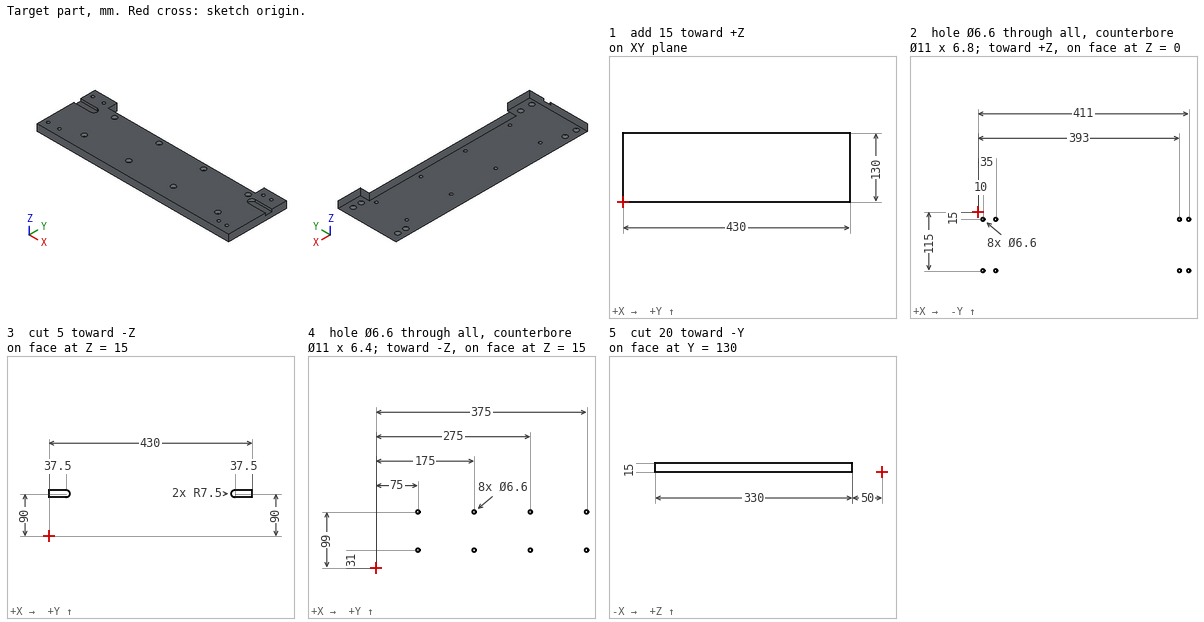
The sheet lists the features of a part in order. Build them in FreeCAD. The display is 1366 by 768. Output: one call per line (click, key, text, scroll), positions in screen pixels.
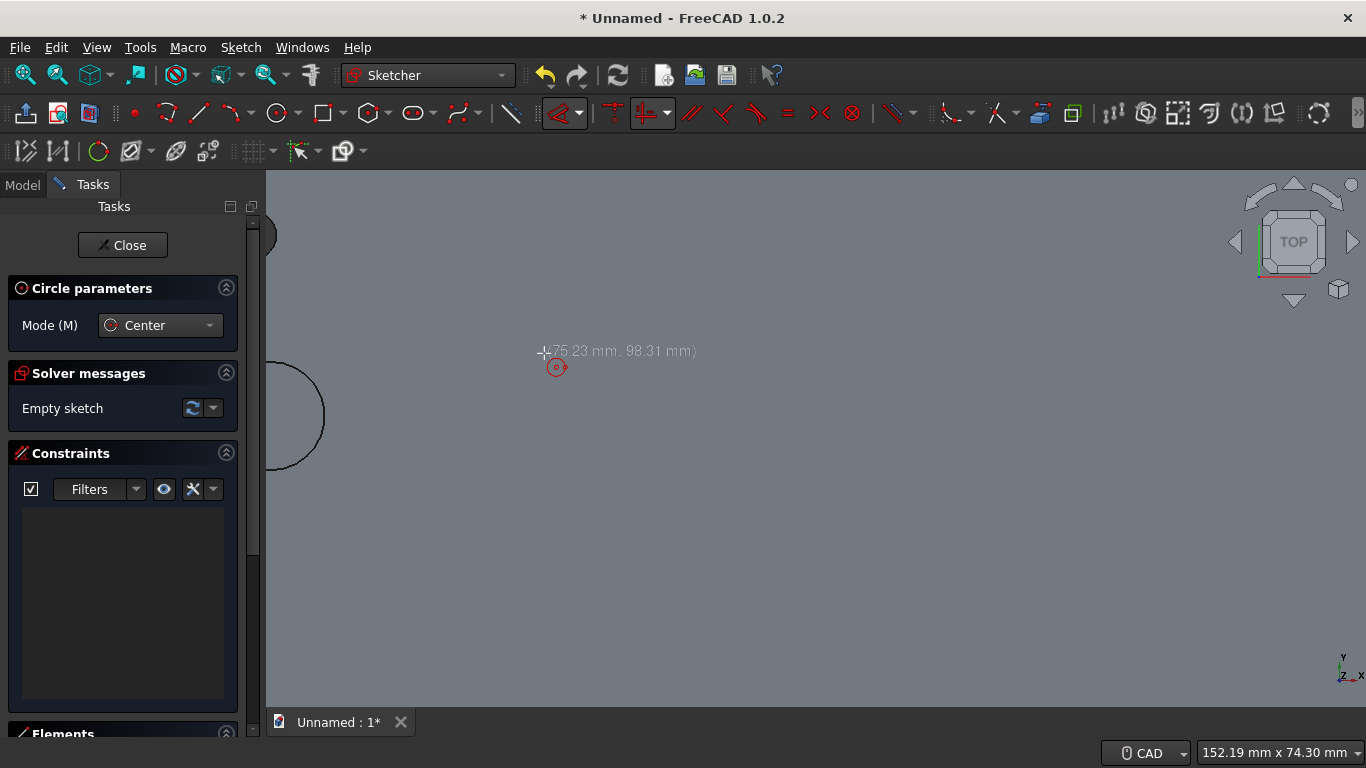
scroll(545, 354, down, 7)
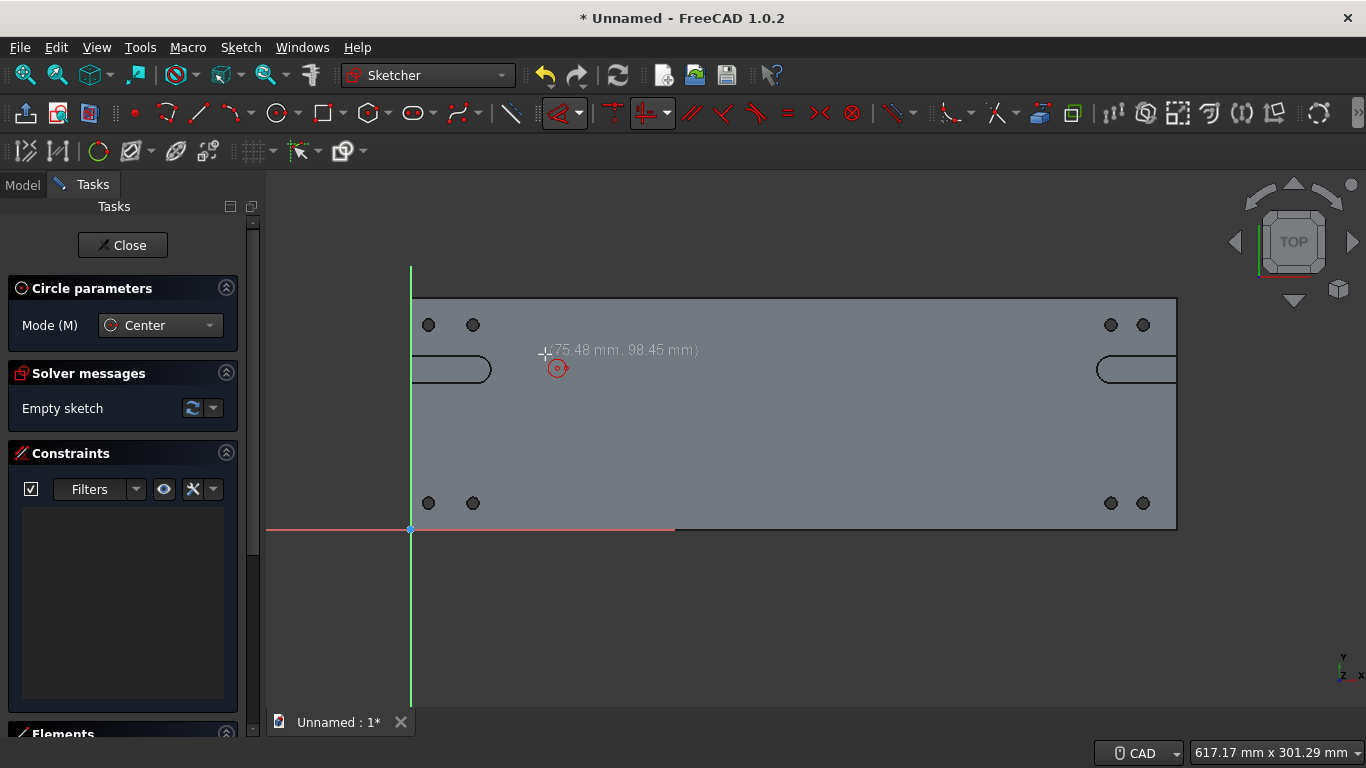
click(544, 354)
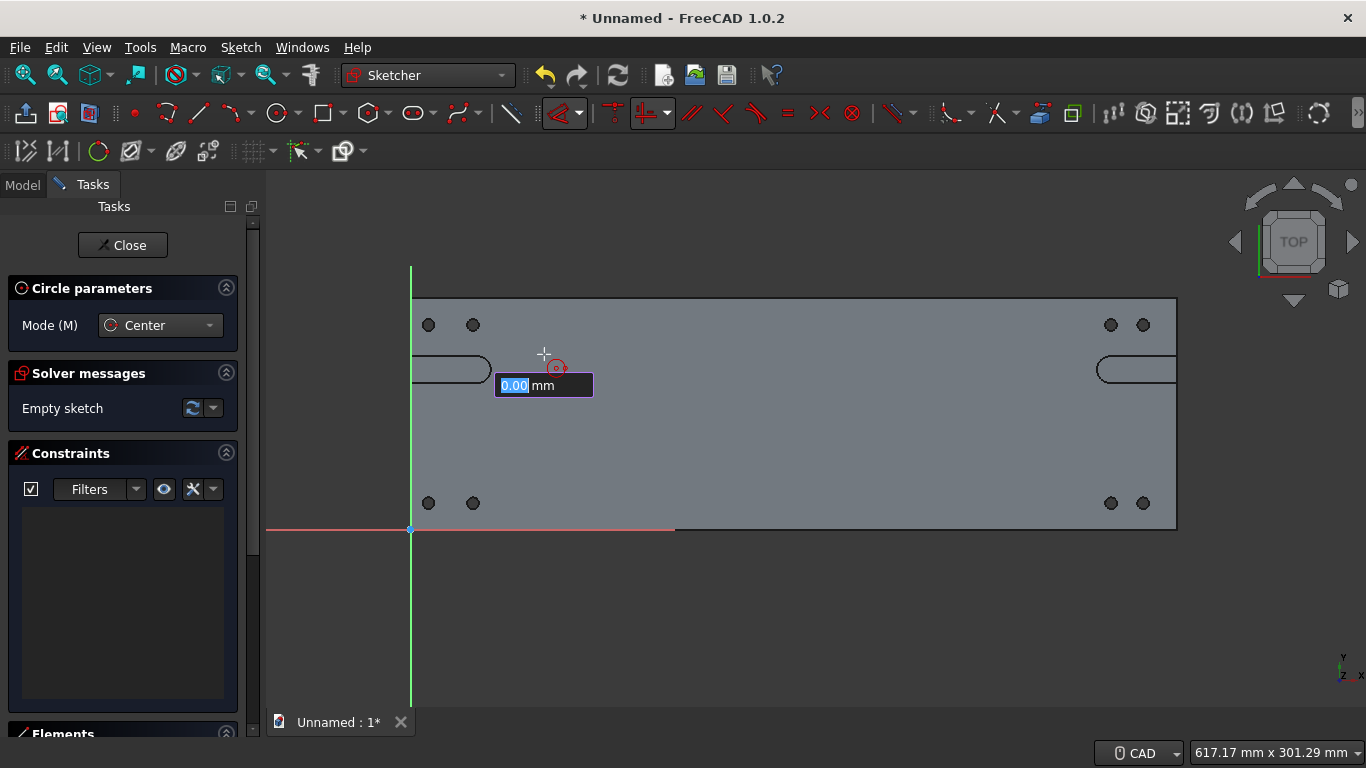
scroll(548, 349, up, 5)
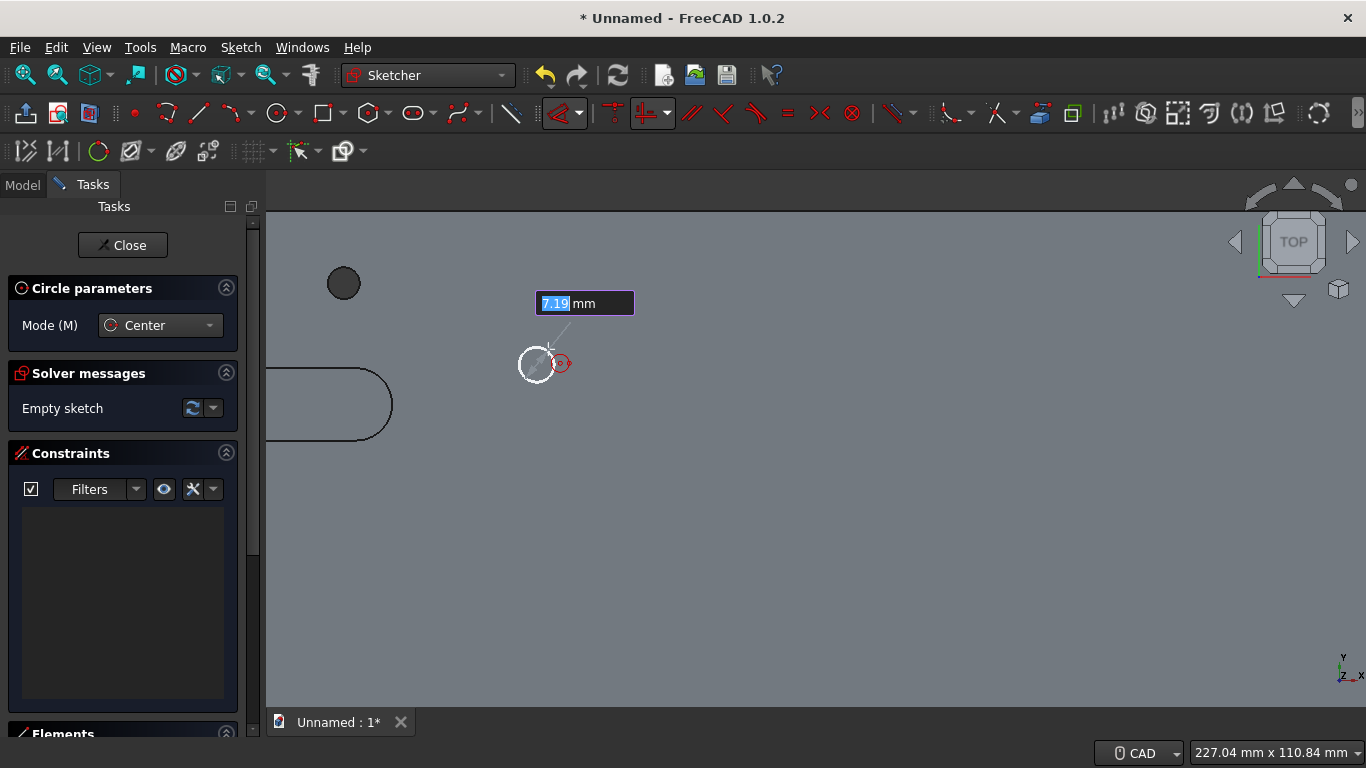
click(549, 349)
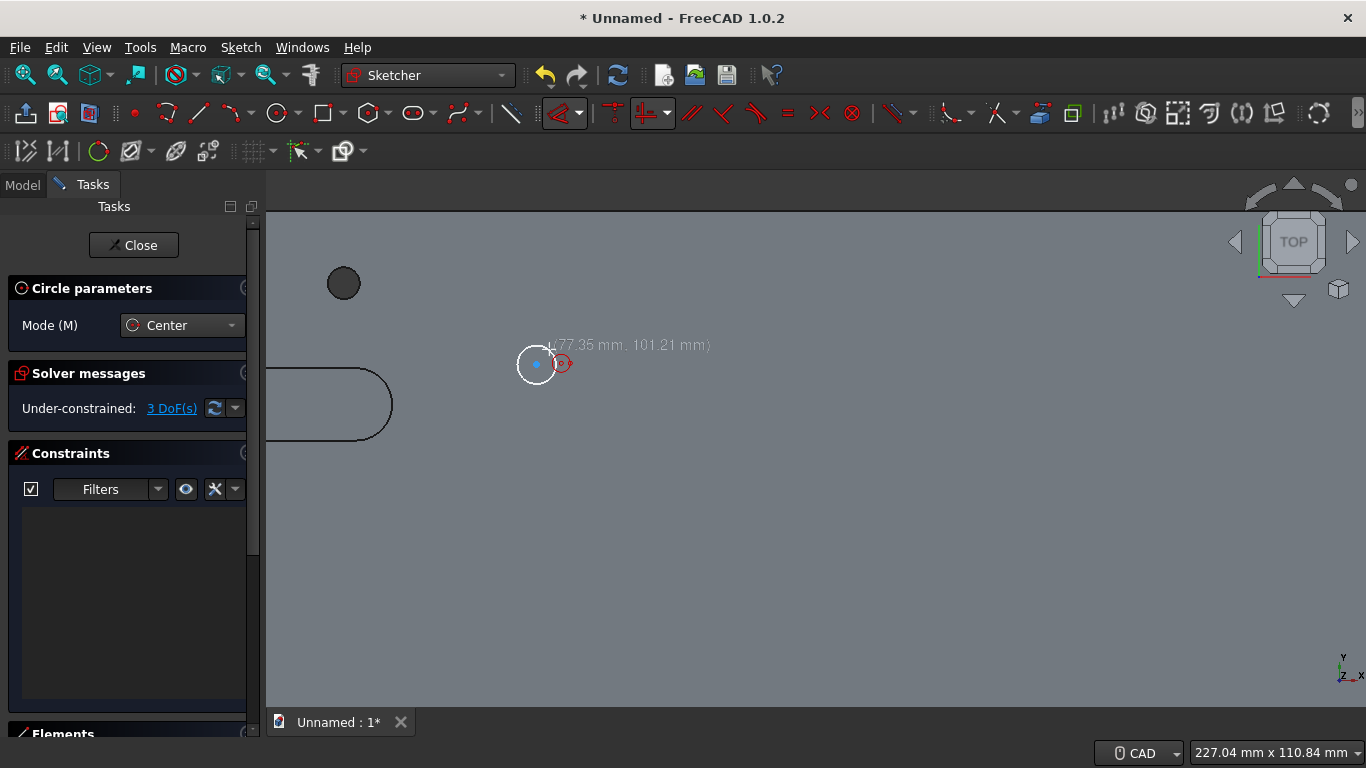
scroll(1022, 361, up, 2)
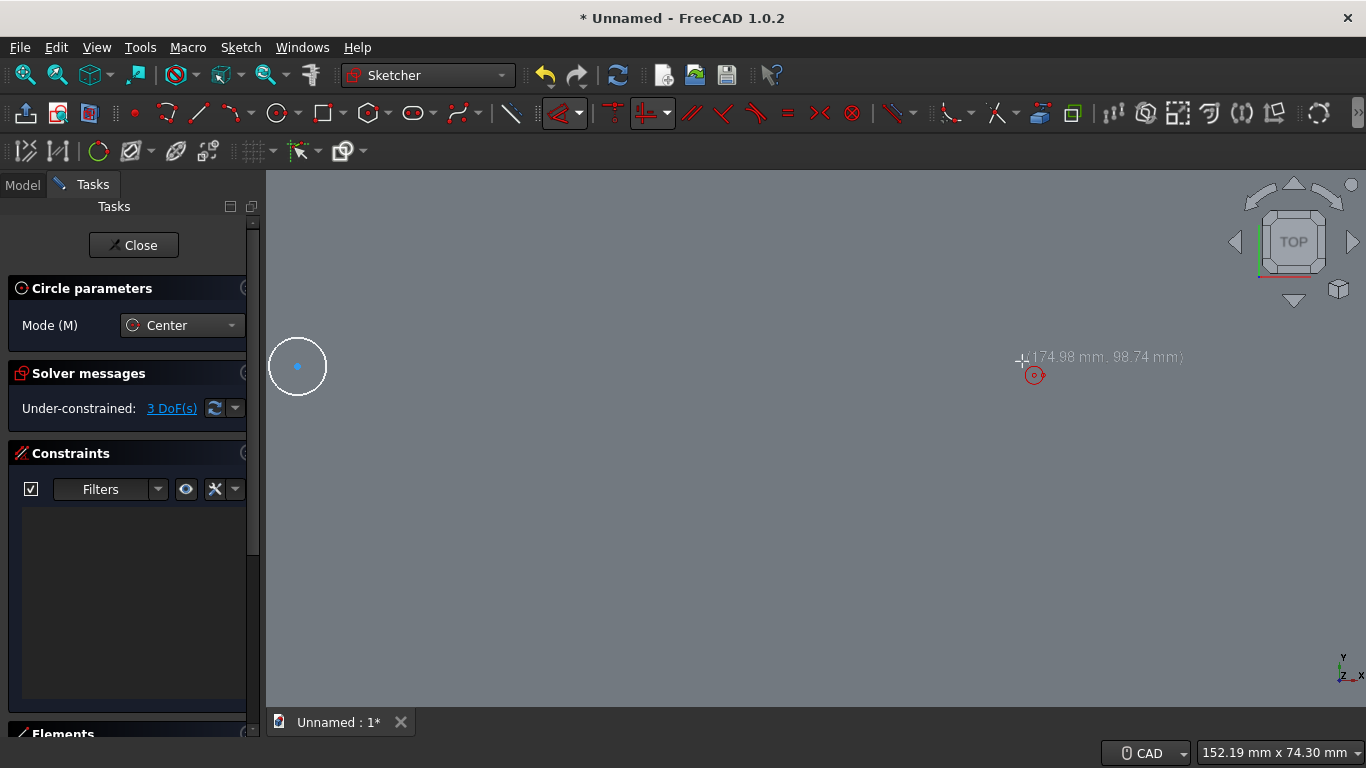
scroll(624, 351, down, 7)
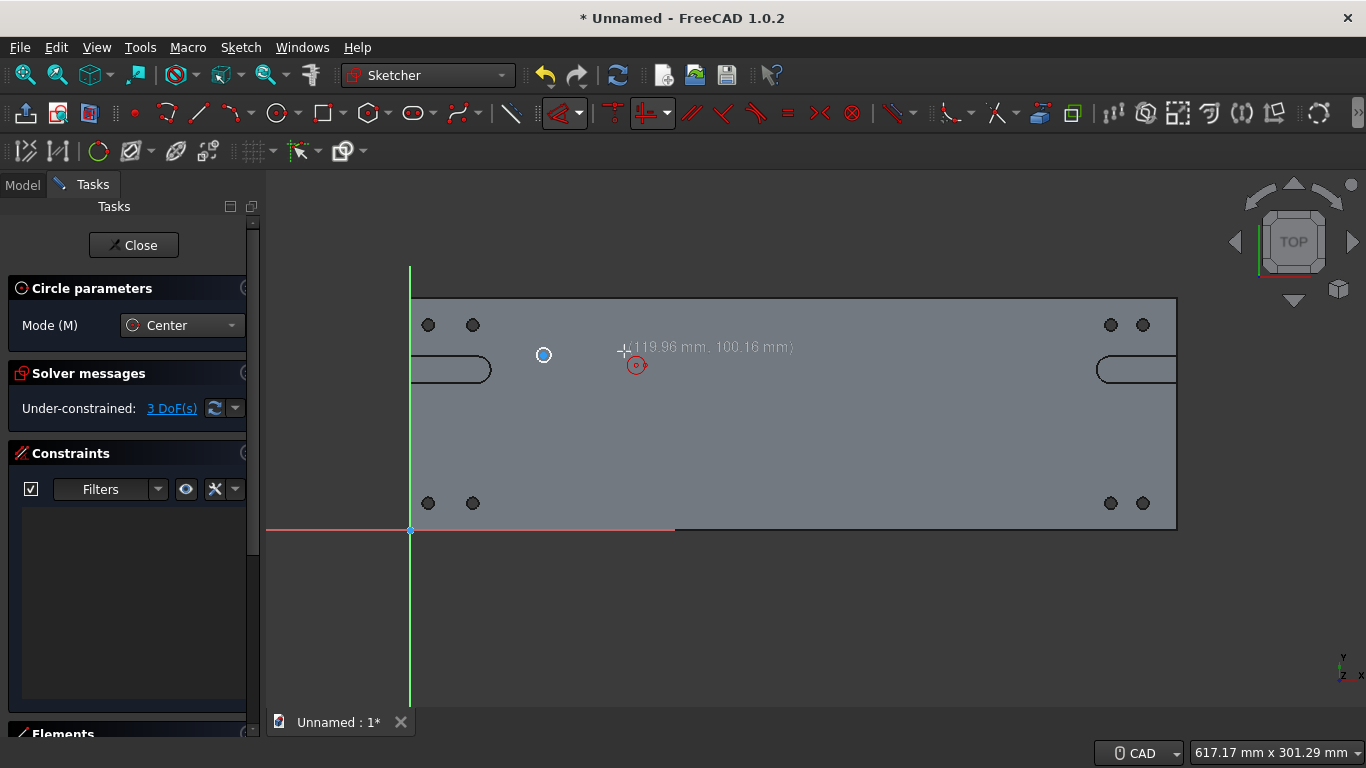
click(722, 354)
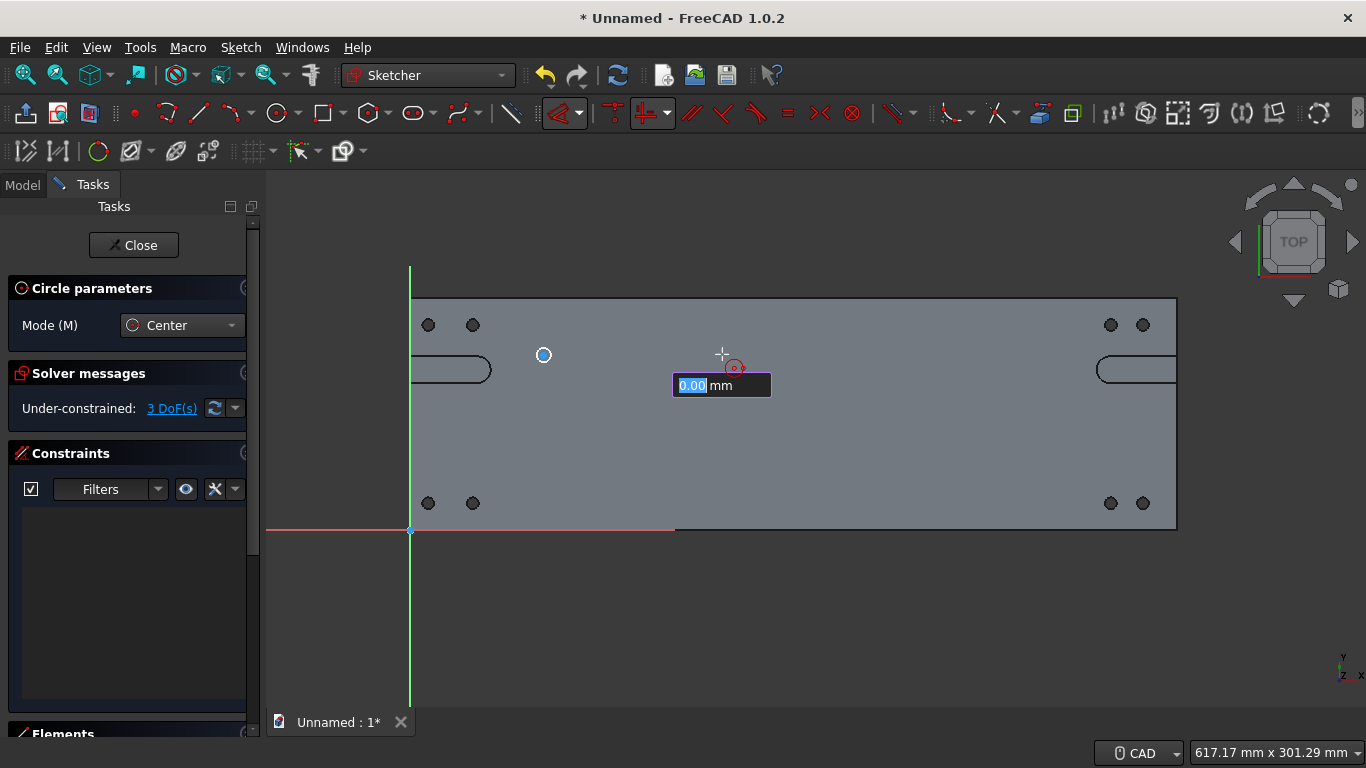
scroll(726, 349, up, 5)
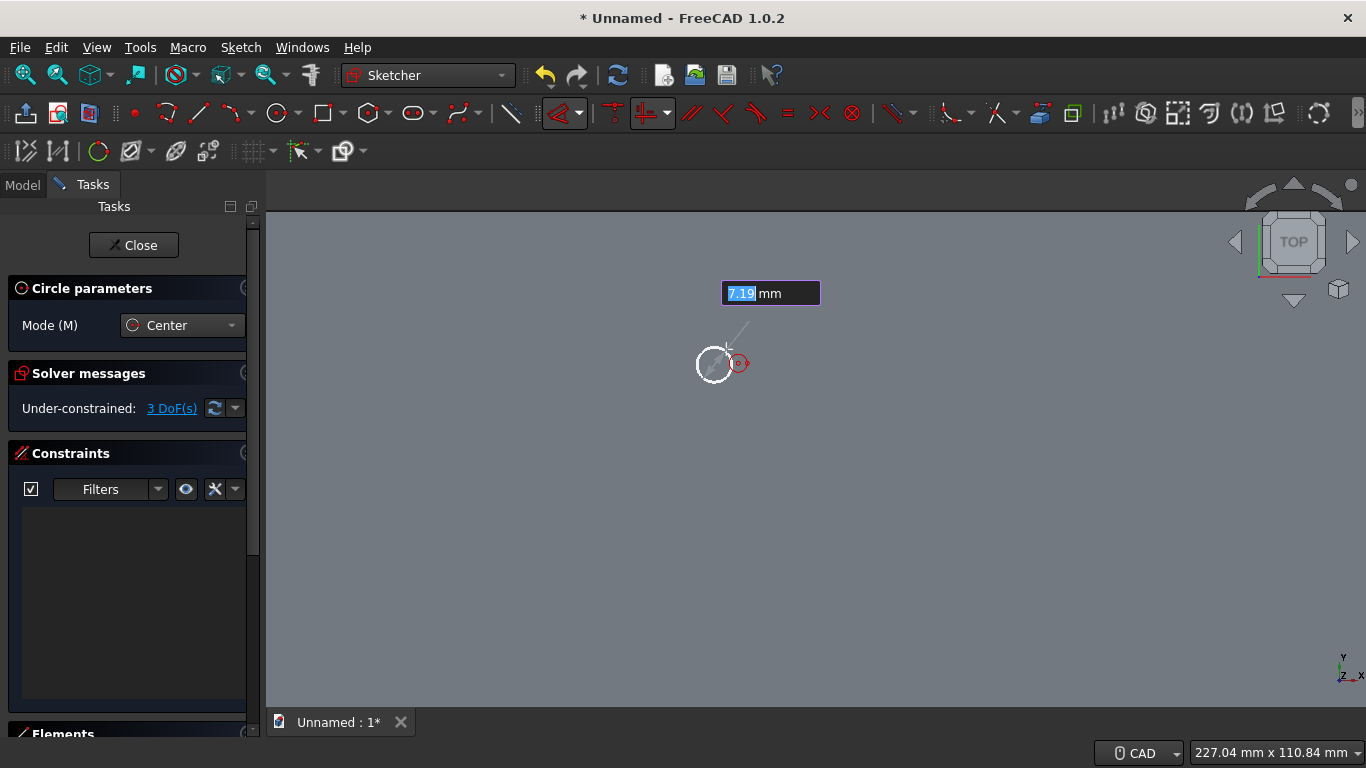
click(727, 350)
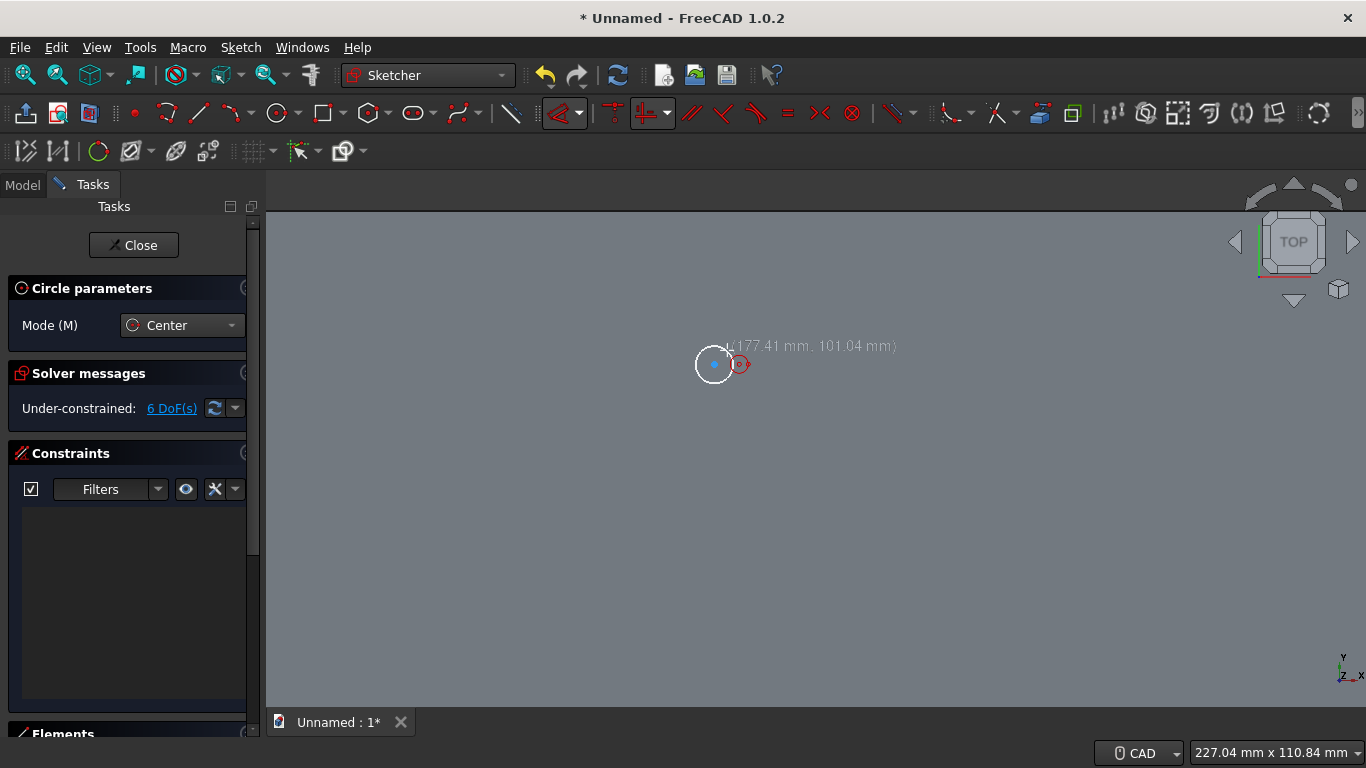
scroll(726, 349, down, 5)